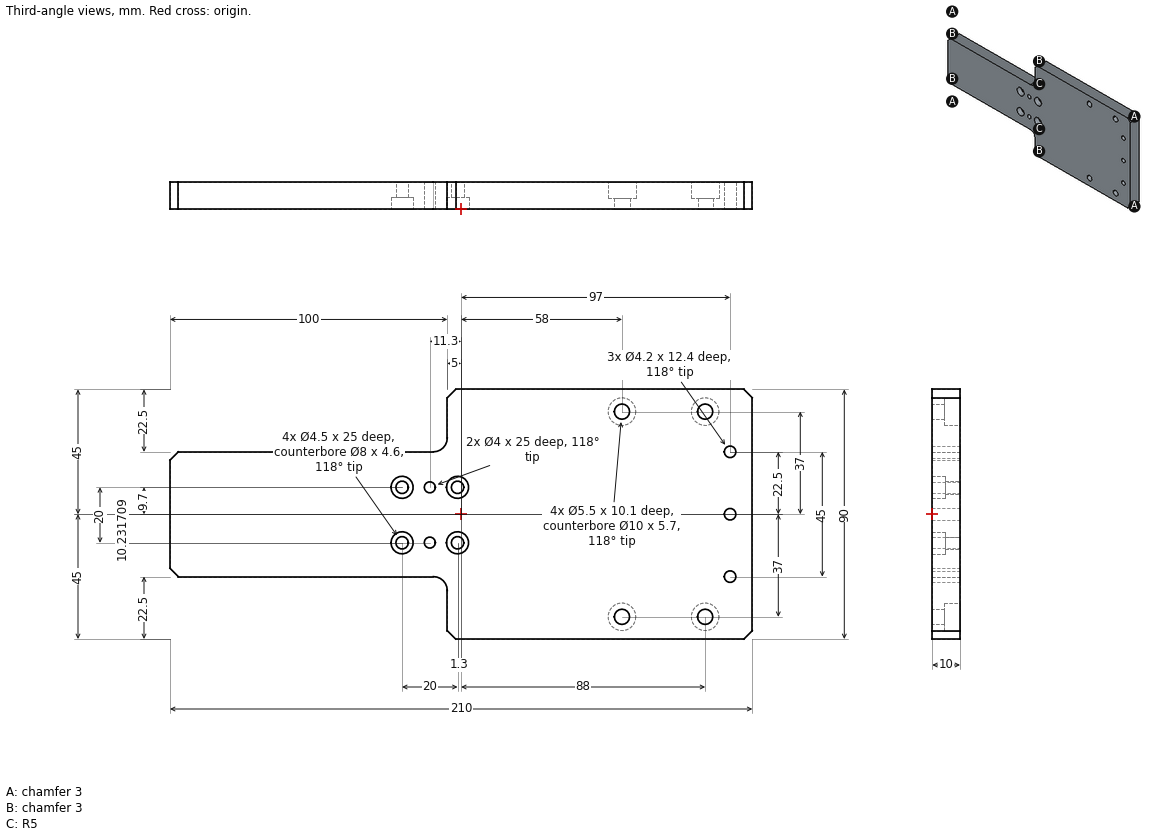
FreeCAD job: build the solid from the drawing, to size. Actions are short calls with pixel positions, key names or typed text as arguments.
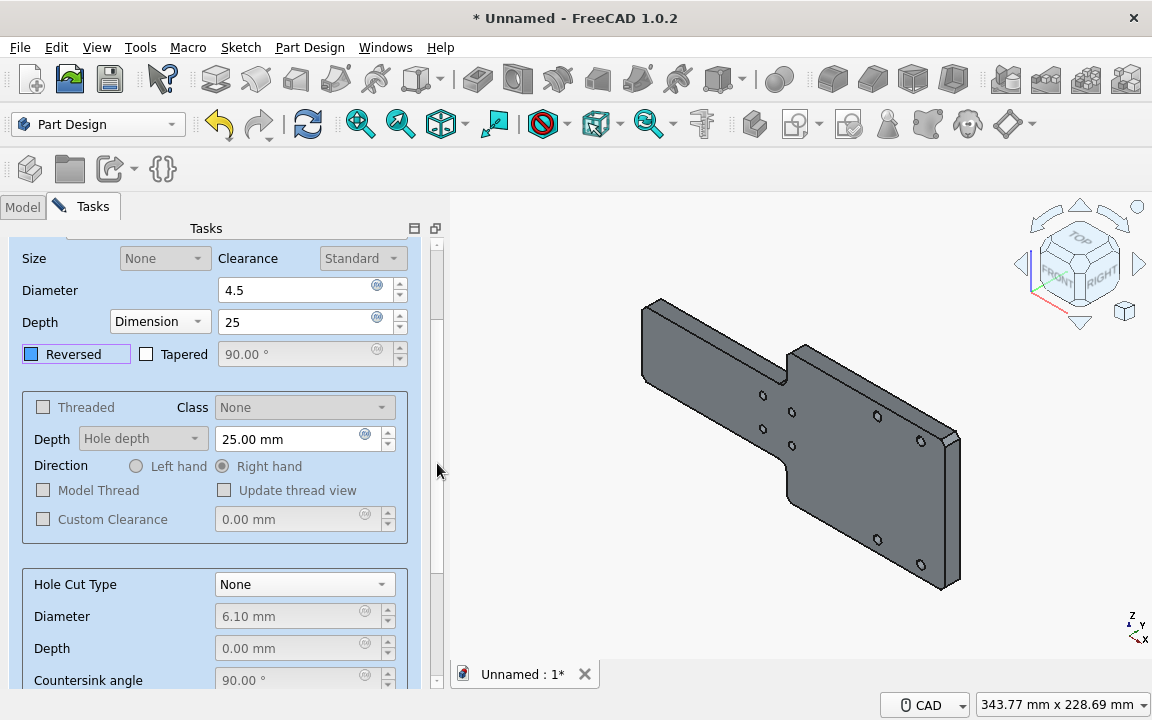
click(306, 584)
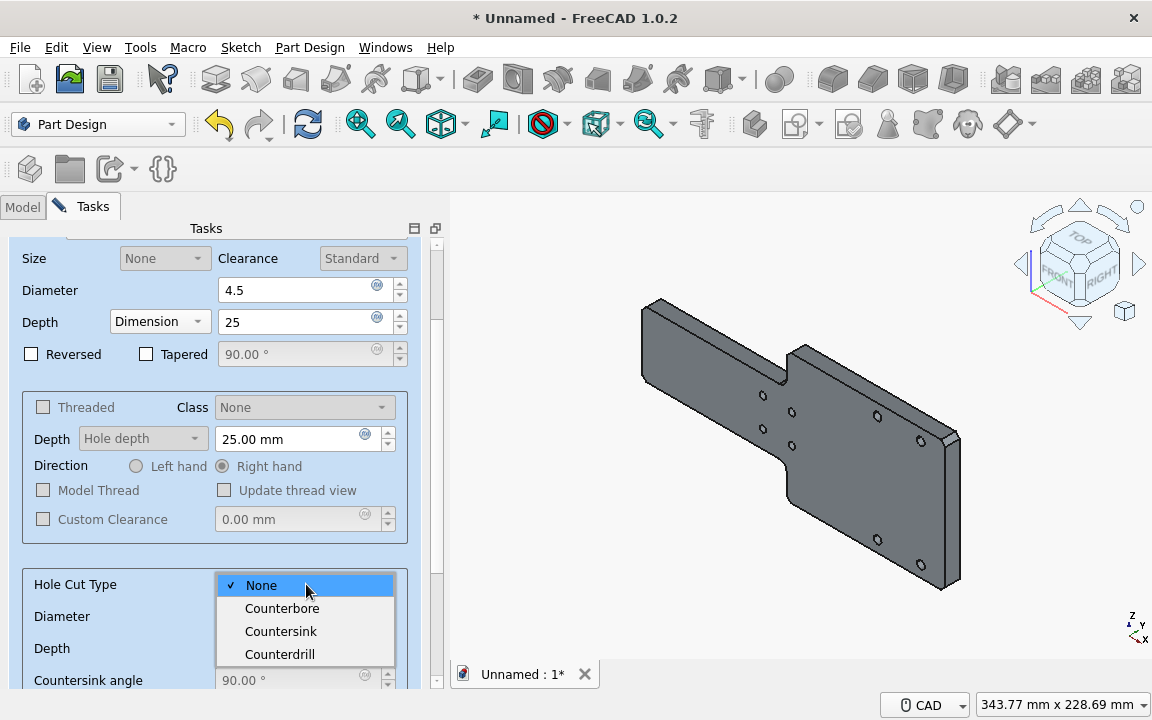
click(304, 608)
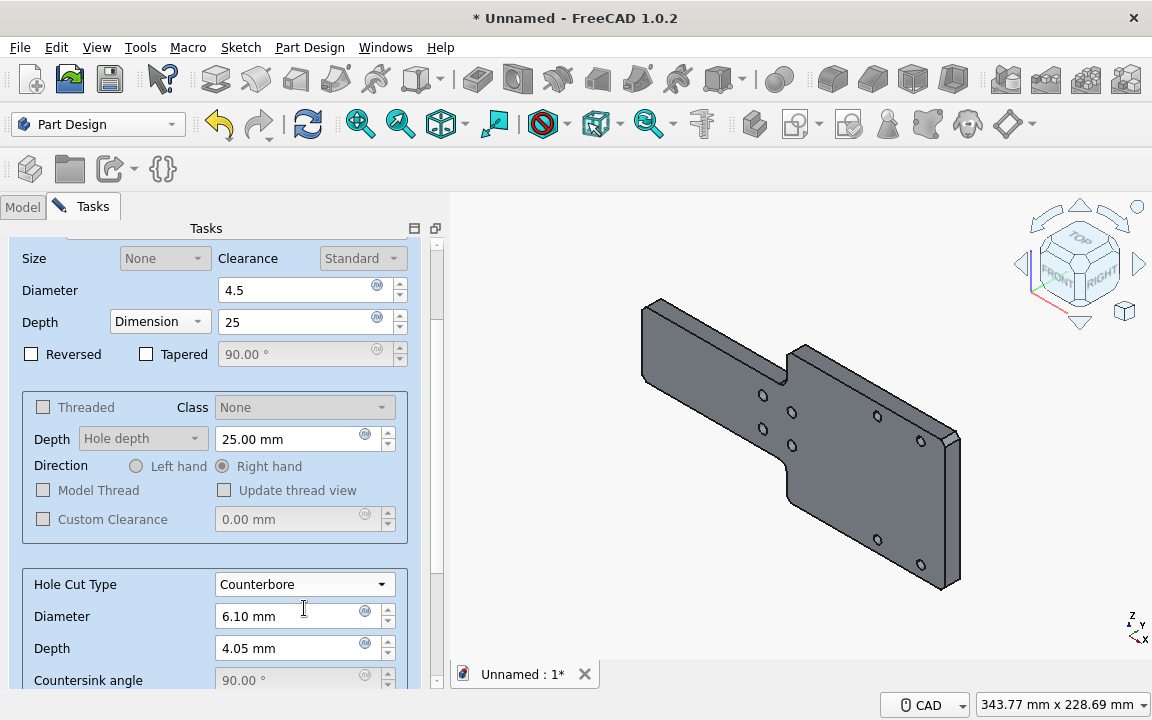
triple_click(298, 616)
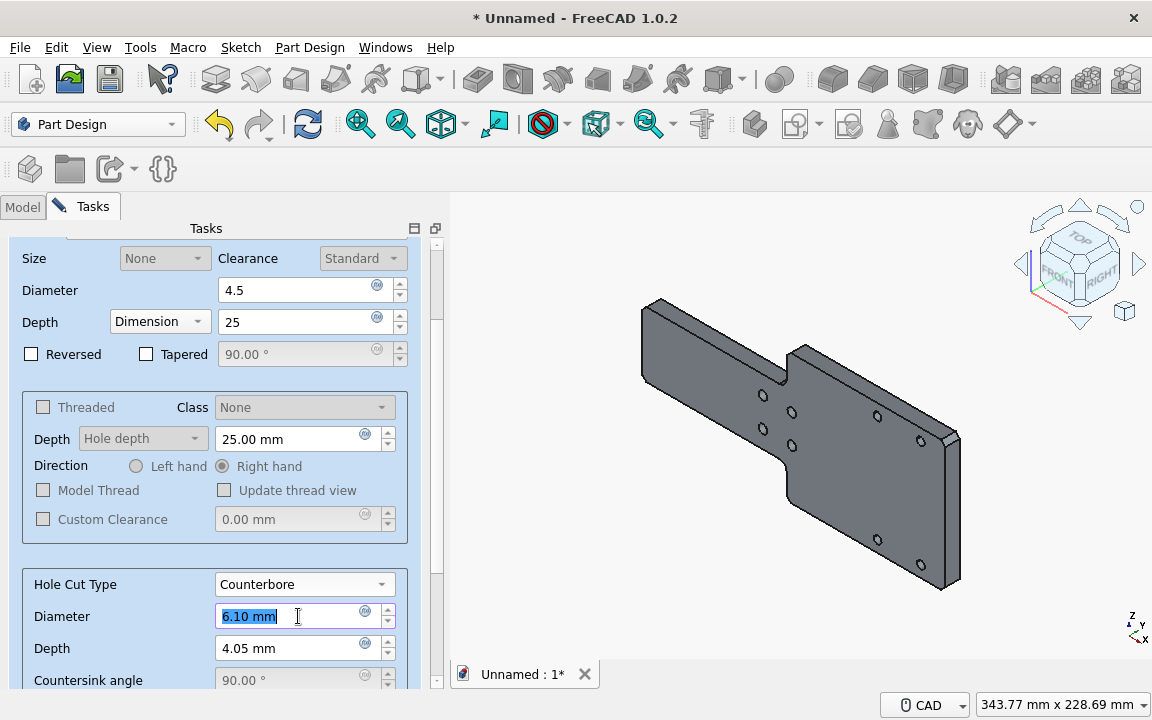
text(8)
key(Tab)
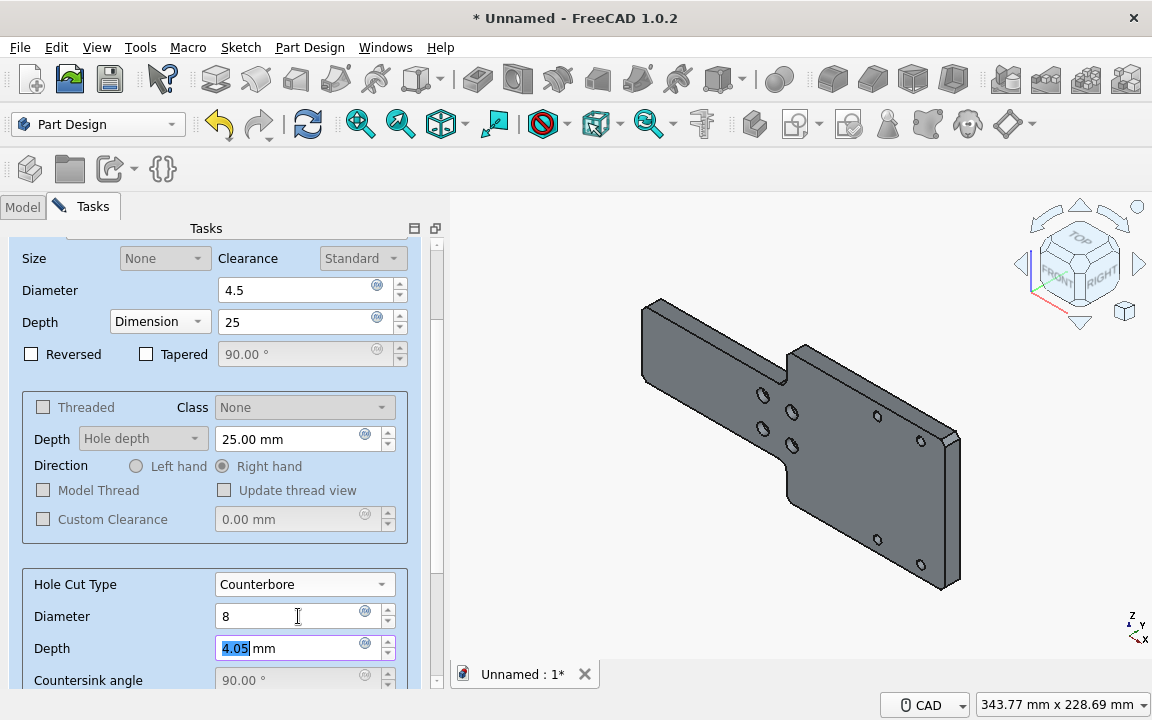
text(4.6)
key(Tab)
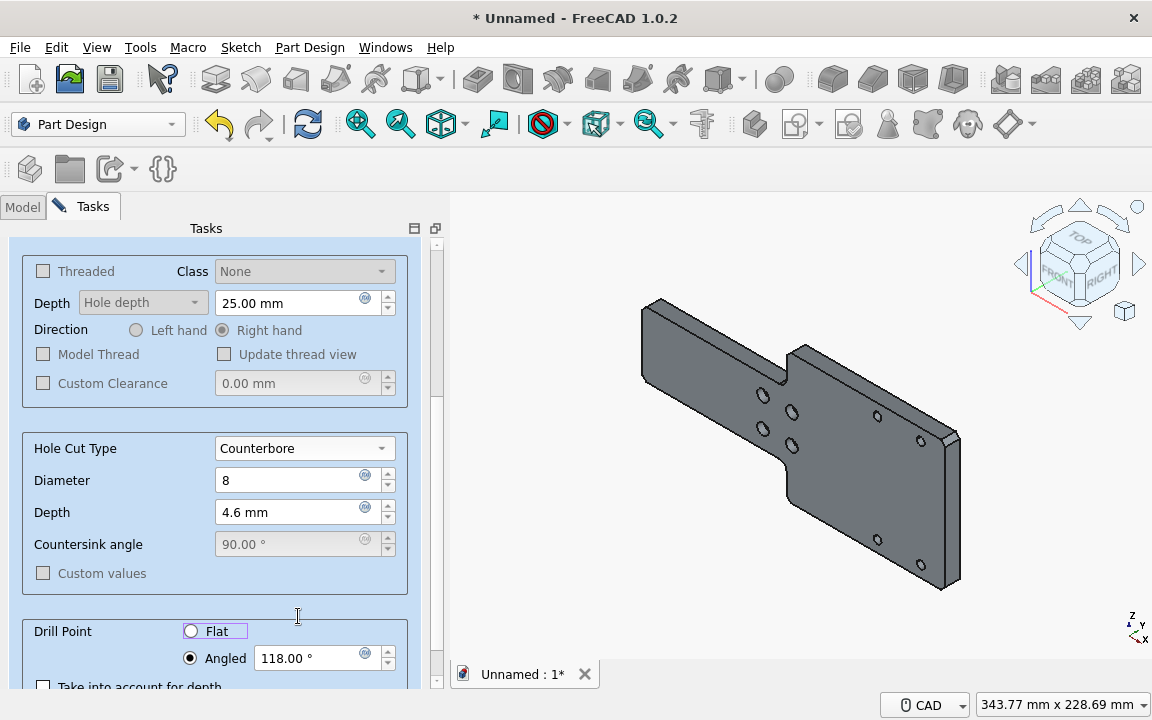
scroll(437, 463, up, 6)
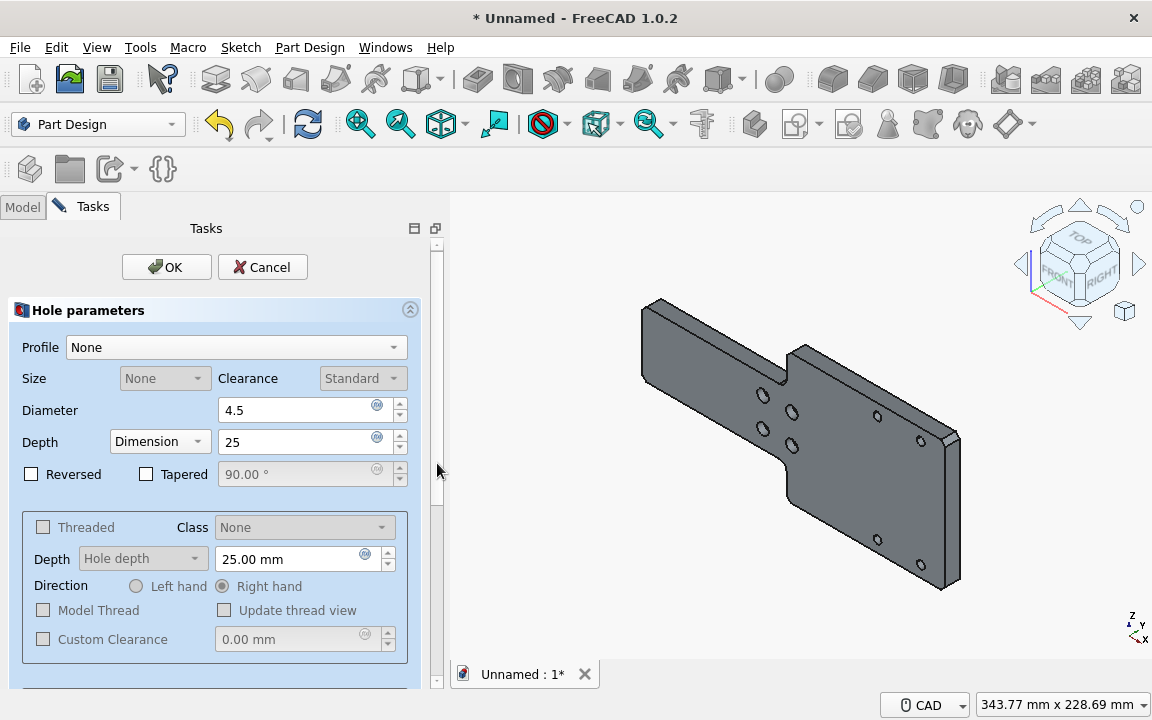
click(167, 267)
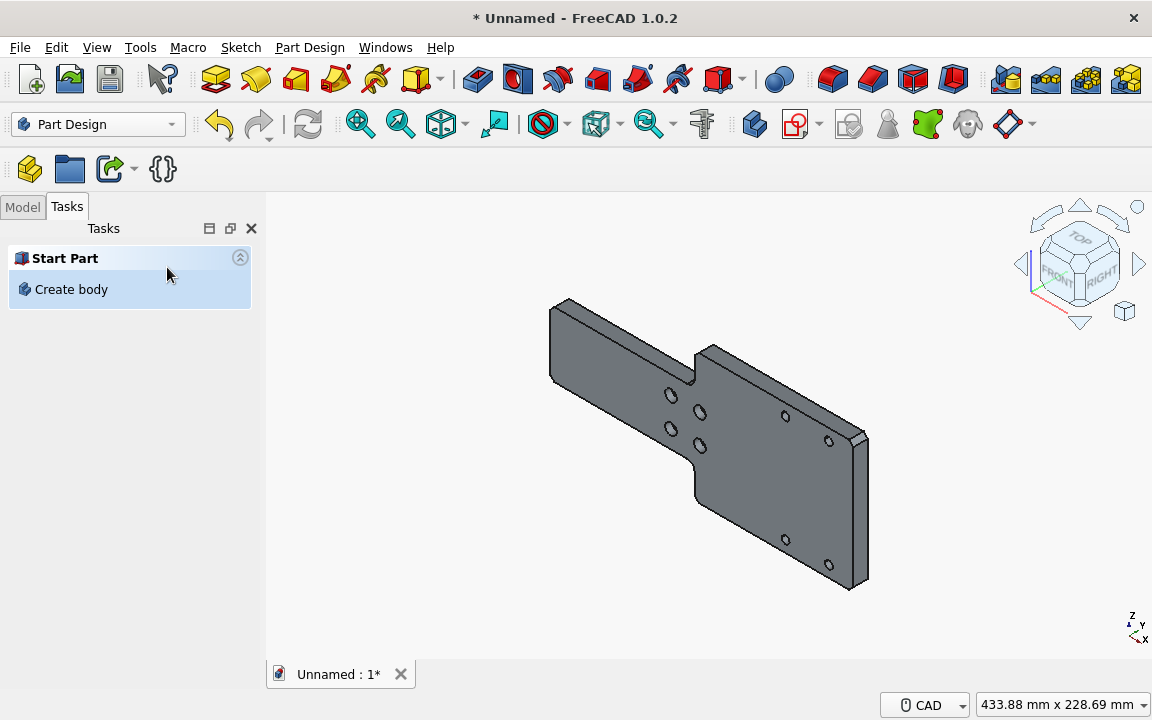
click(796, 124)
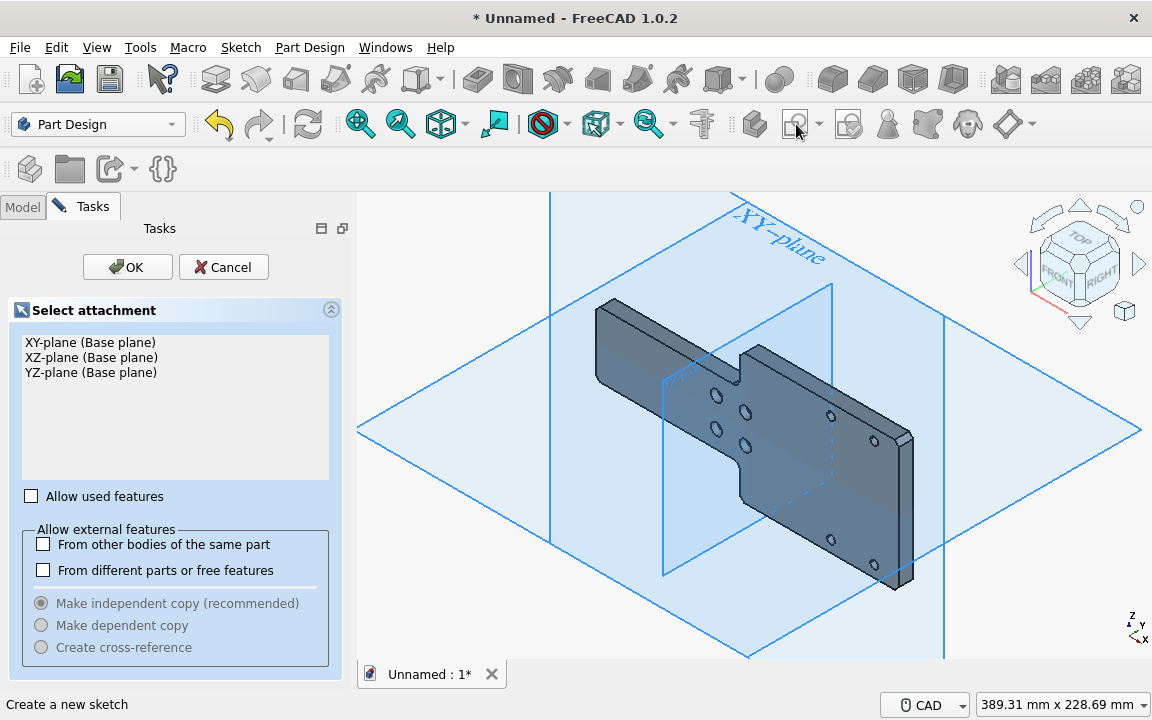
click(82, 358)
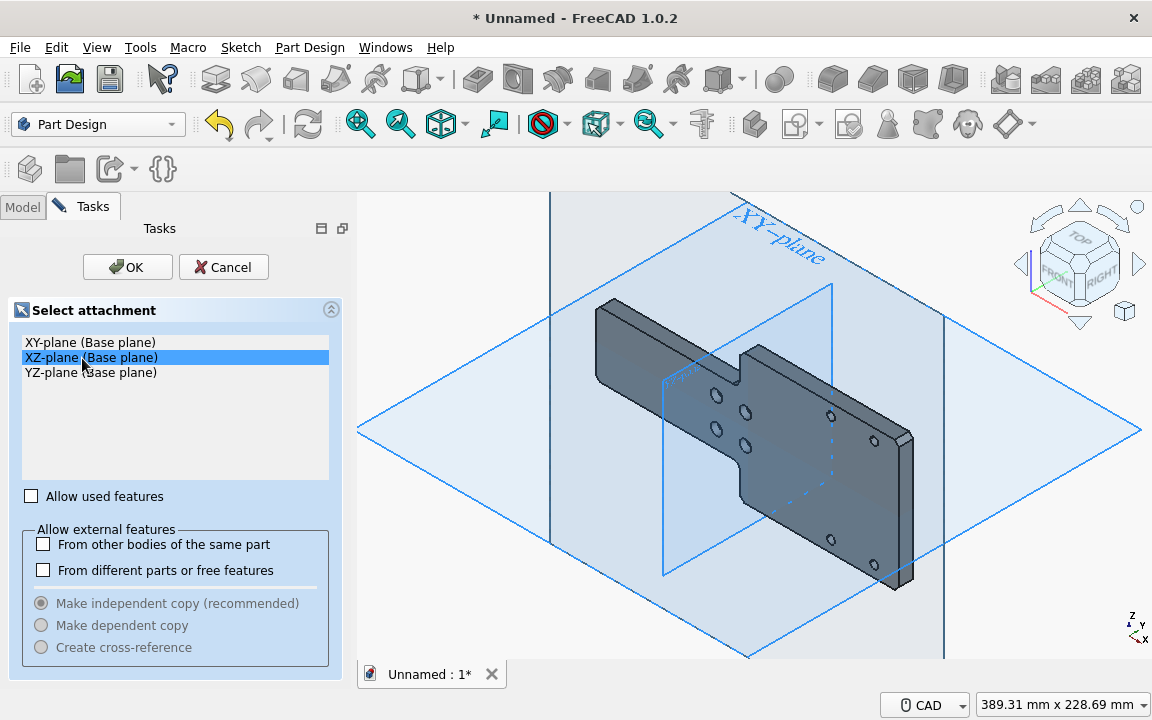
click(128, 267)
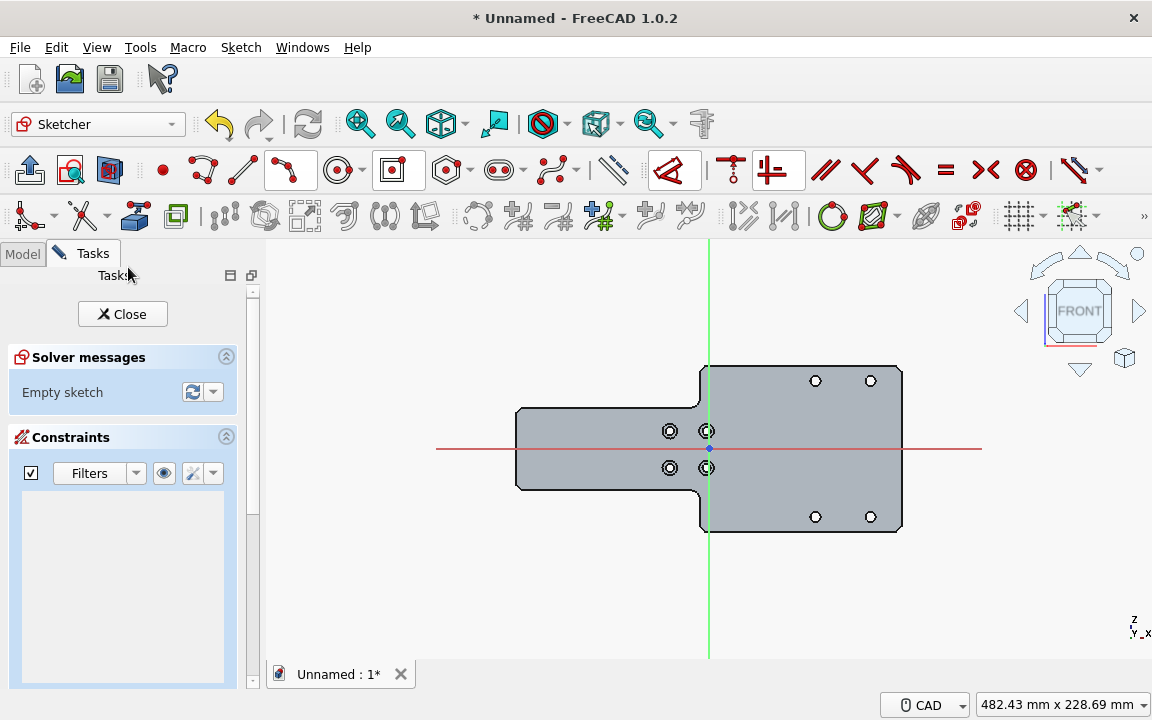
scroll(708, 450, up, 9)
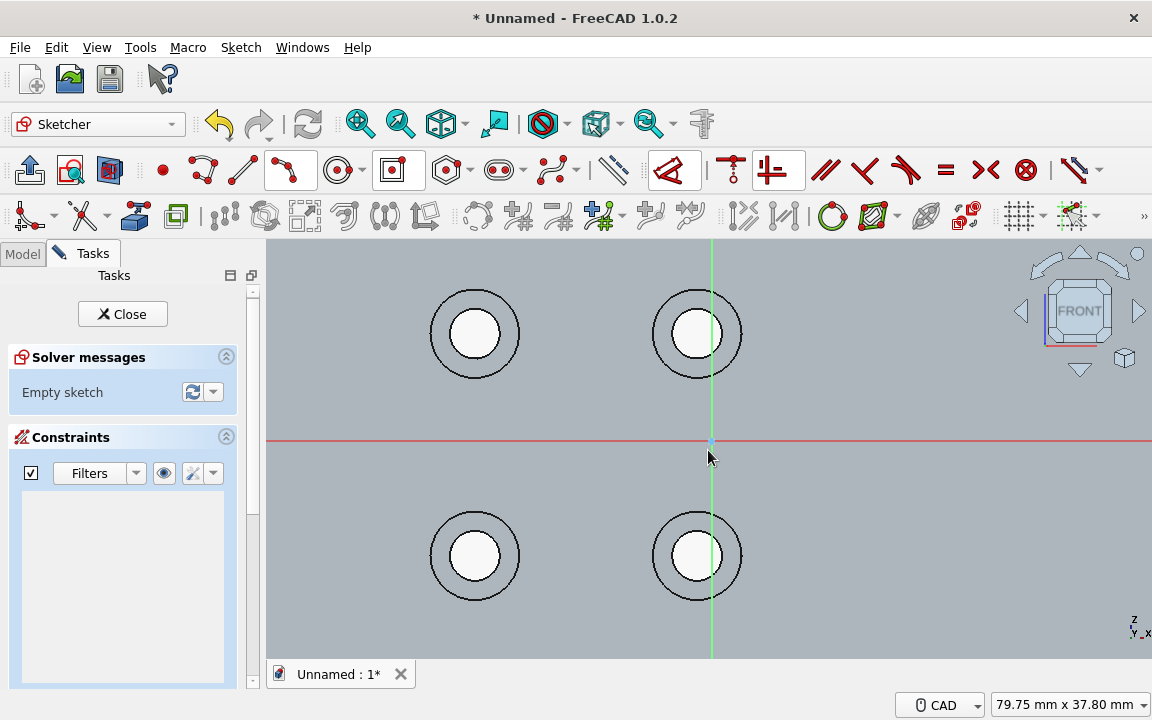
click(338, 170)